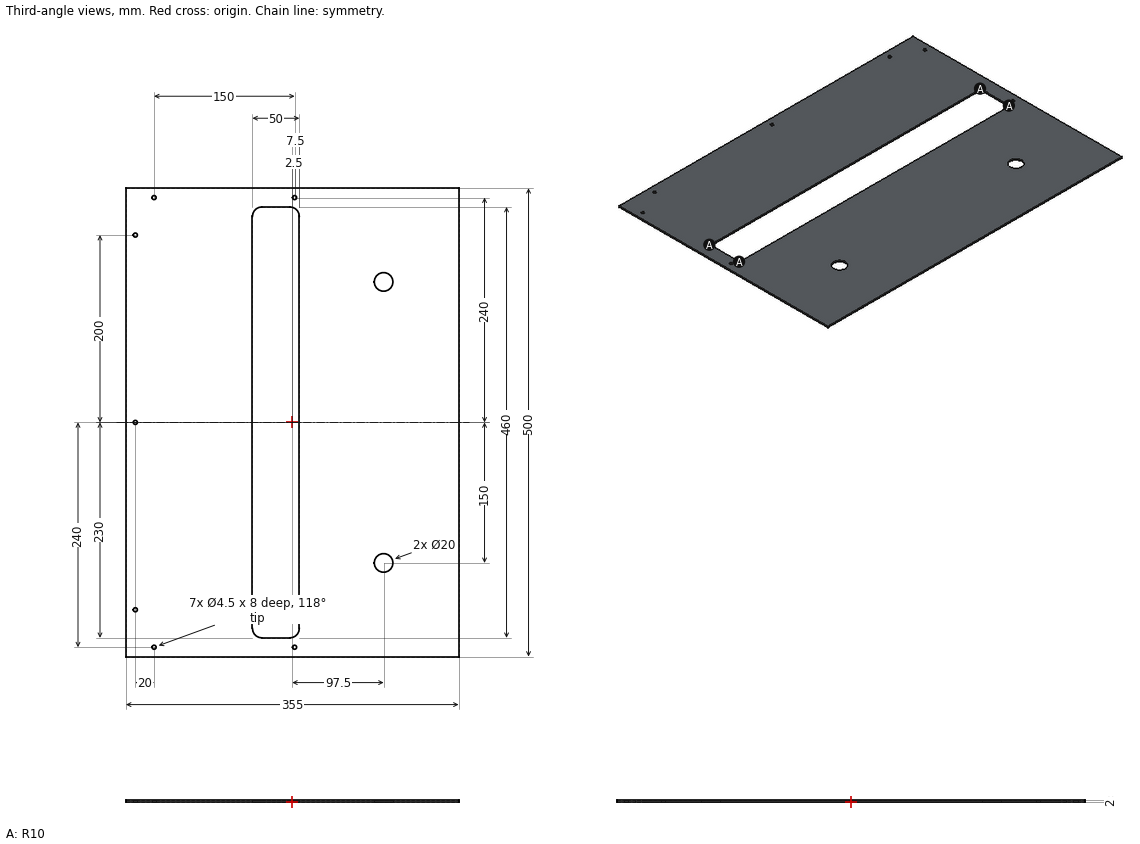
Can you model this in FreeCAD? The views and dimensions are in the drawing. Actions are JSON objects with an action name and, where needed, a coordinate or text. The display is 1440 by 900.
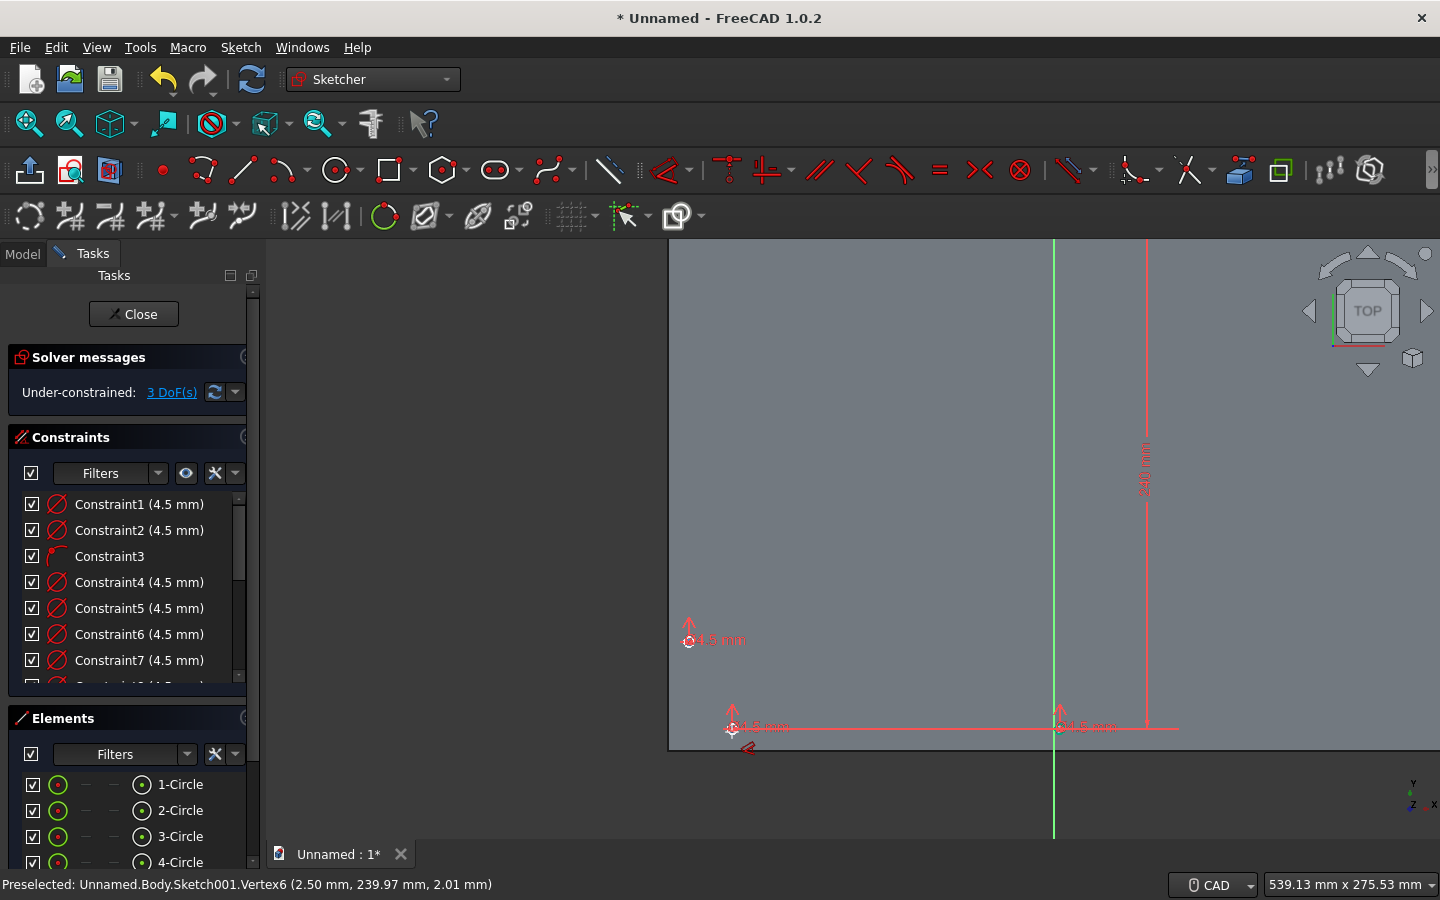
{"action": "left_click", "coordinate": [732, 729]}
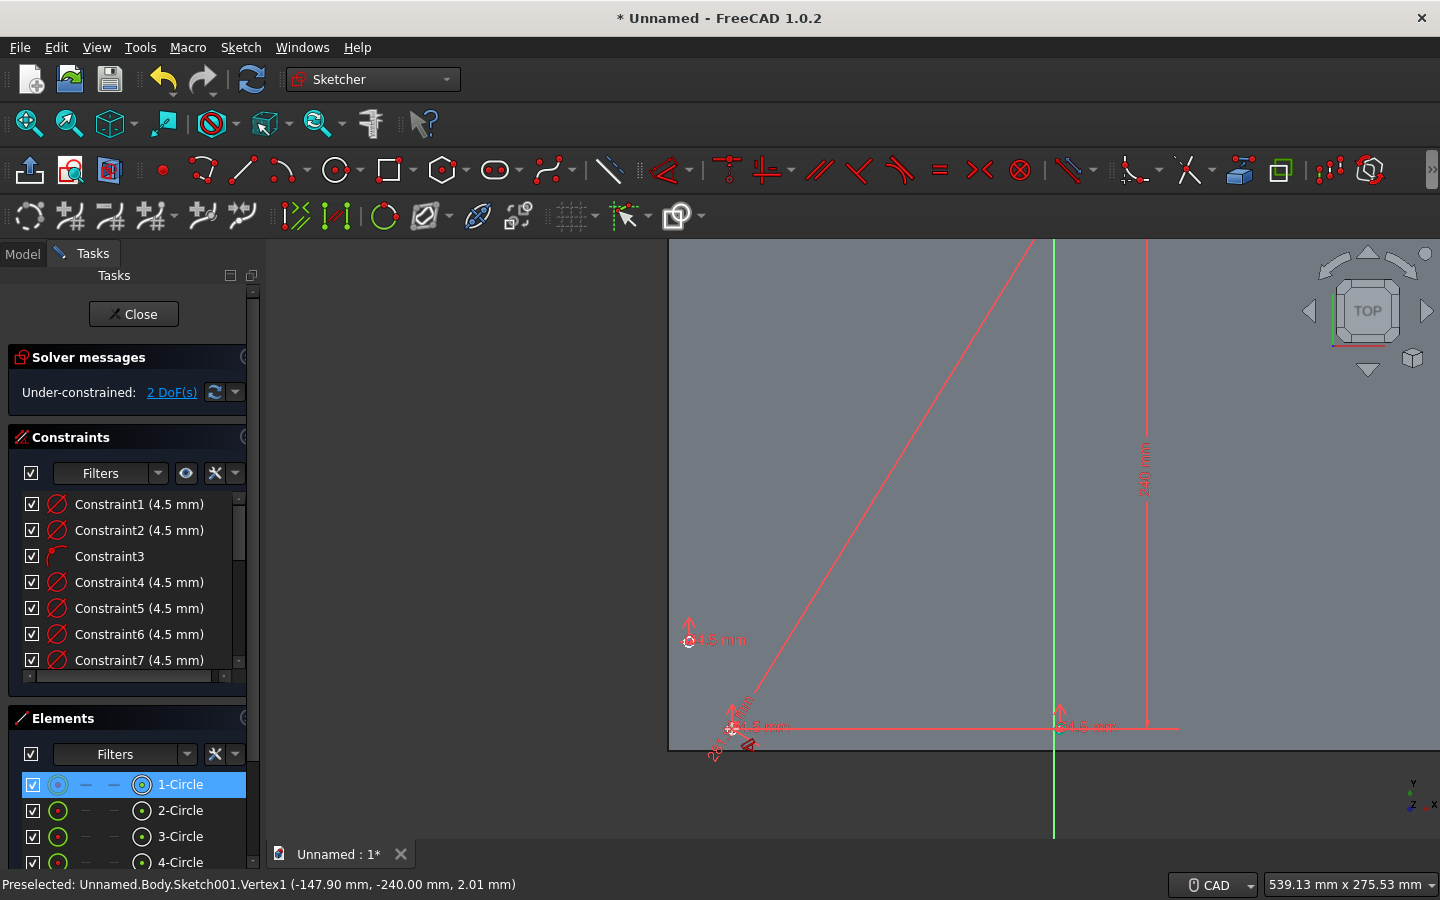
{"action": "scroll", "coordinate": [732, 732], "scroll_direction": "down", "scroll_amount": 5}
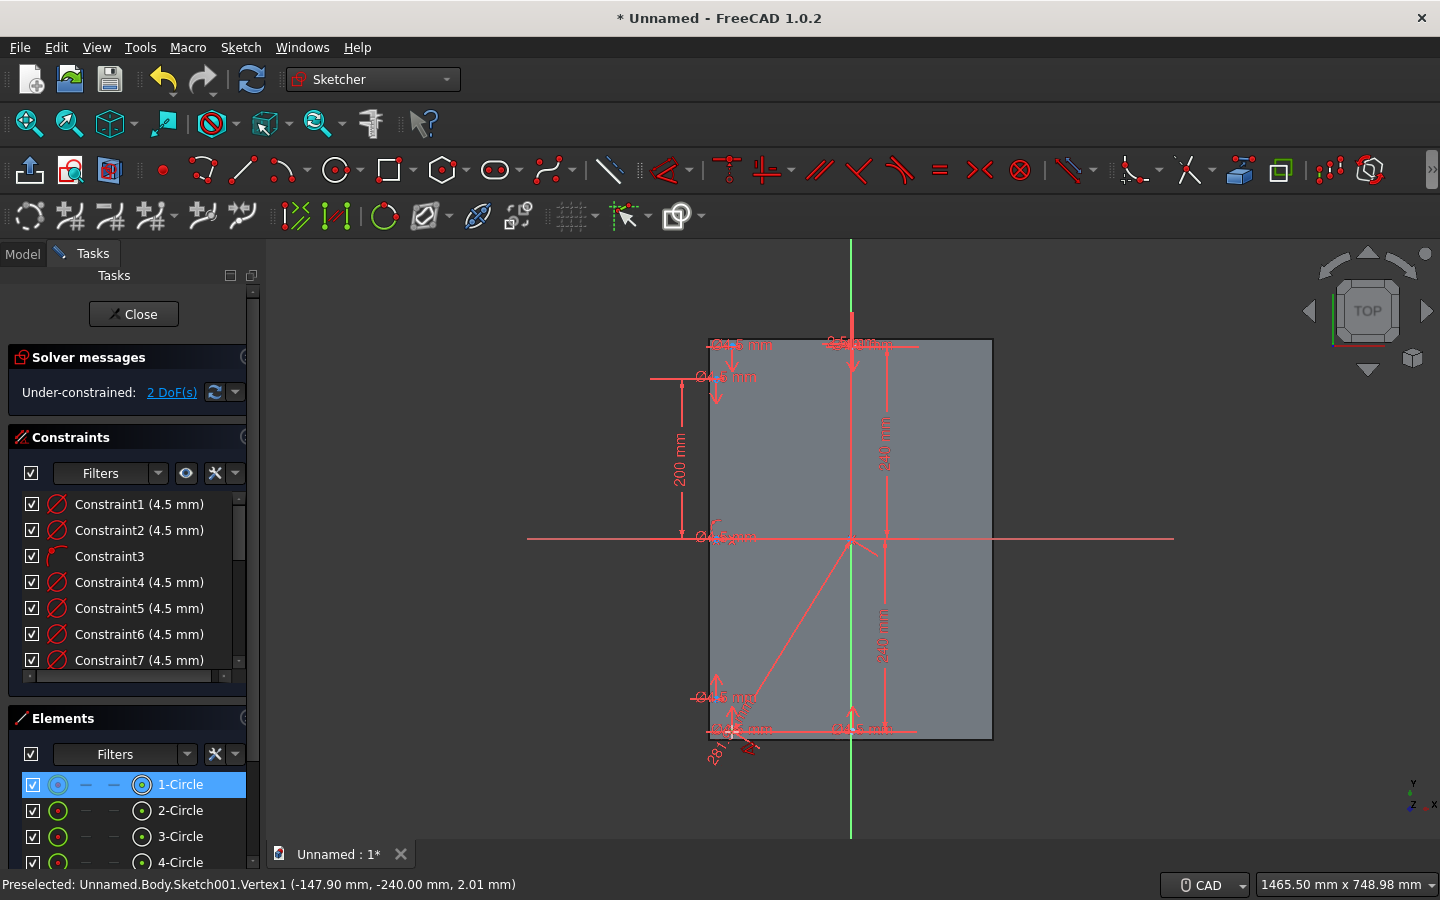
{"action": "scroll", "coordinate": [716, 539], "scroll_direction": "up", "scroll_amount": 5}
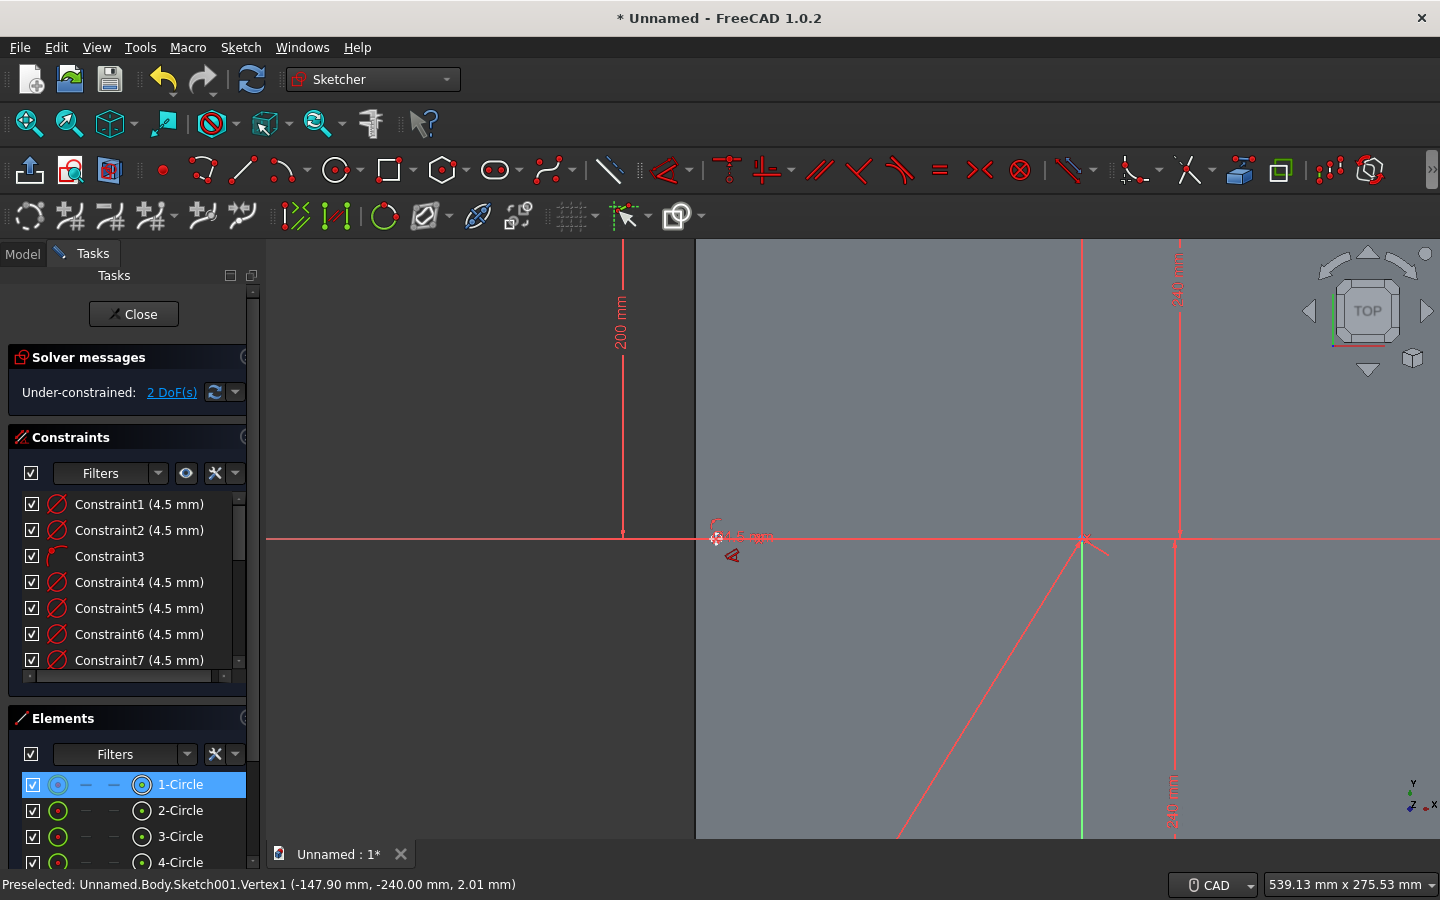
{"action": "left_click", "coordinate": [717, 539]}
{"action": "left_click", "coordinate": [738, 505]}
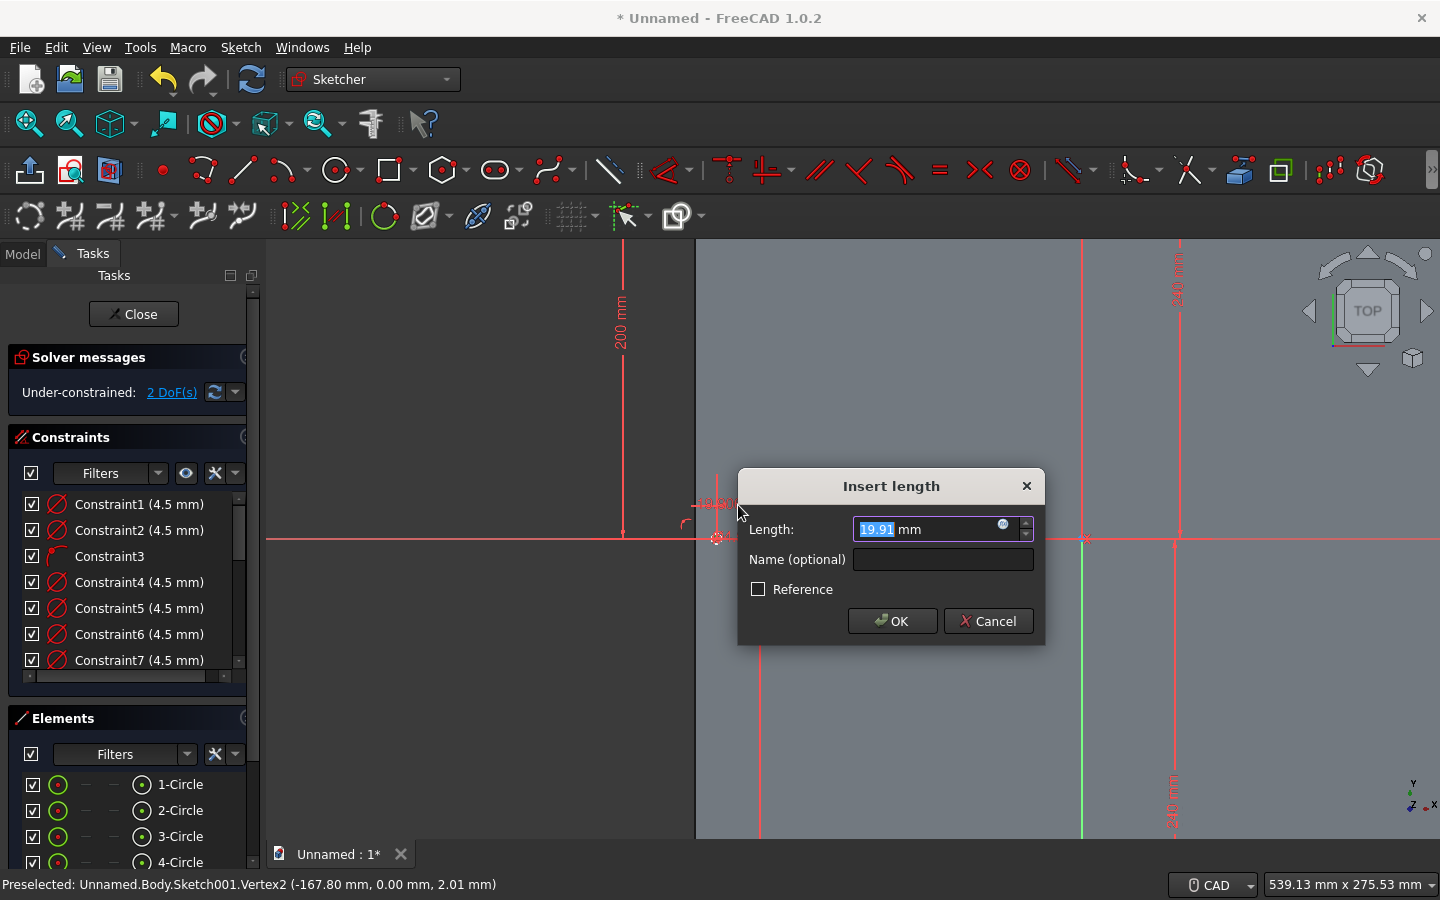
{"action": "type", "text": "20"}
{"action": "key", "text": "Return"}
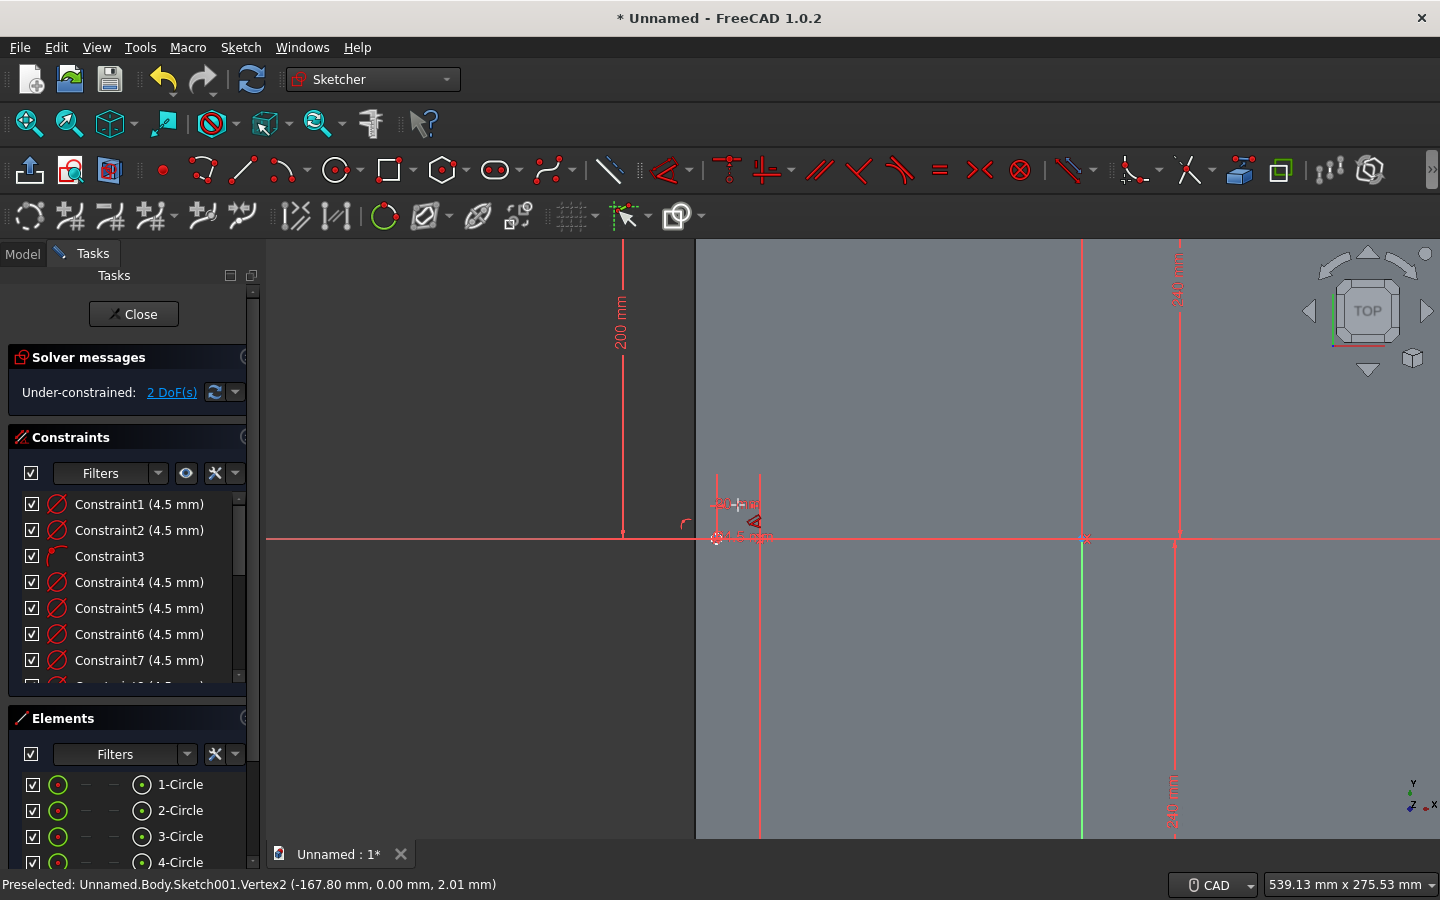
{"action": "scroll", "coordinate": [716, 539], "scroll_direction": "down", "scroll_amount": 5}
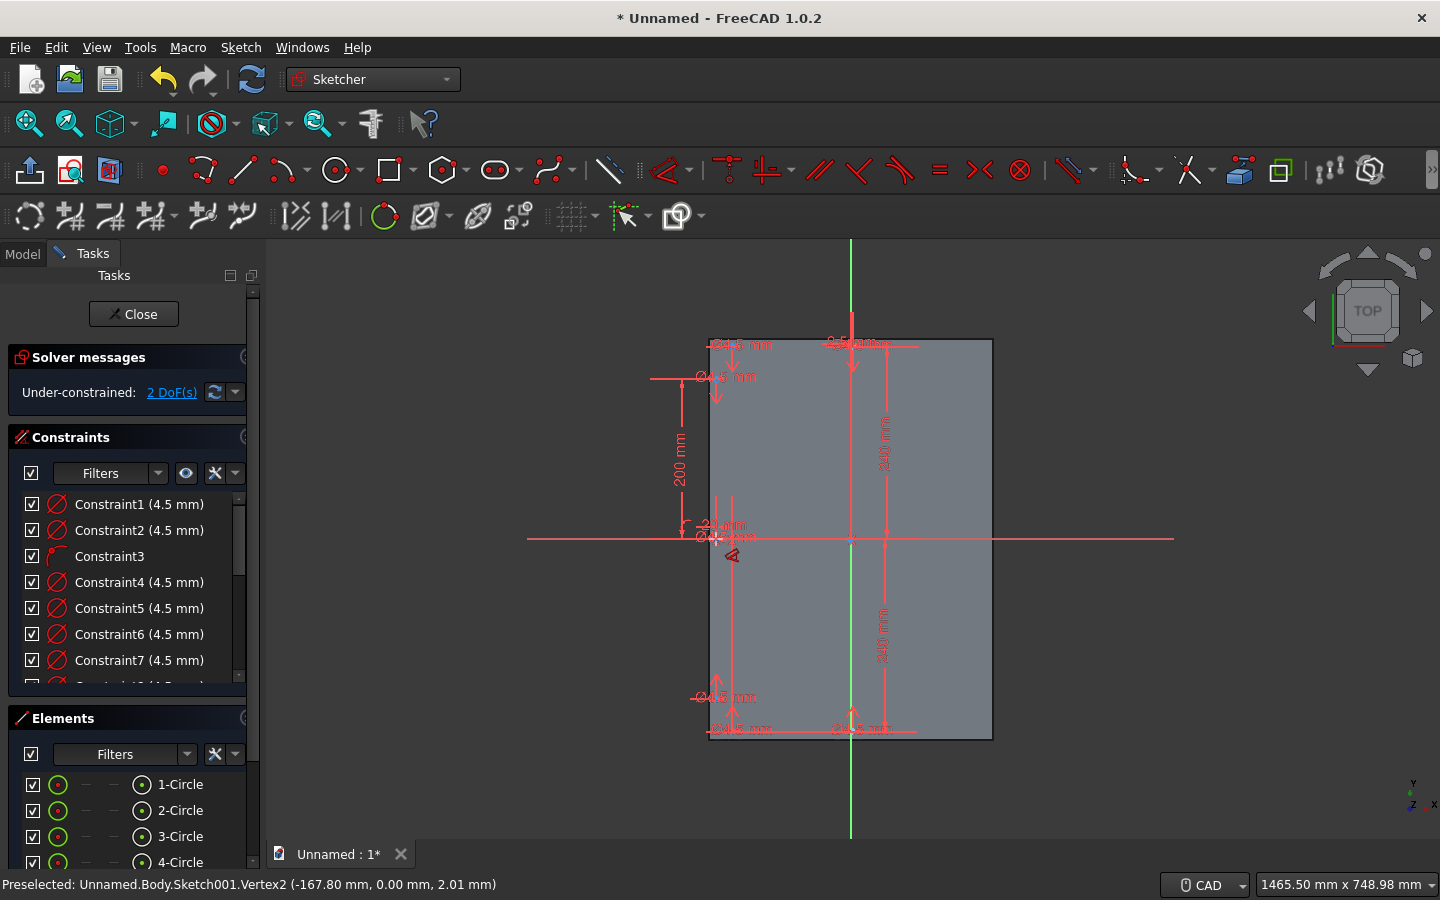
{"action": "scroll", "coordinate": [732, 732], "scroll_direction": "up", "scroll_amount": 5}